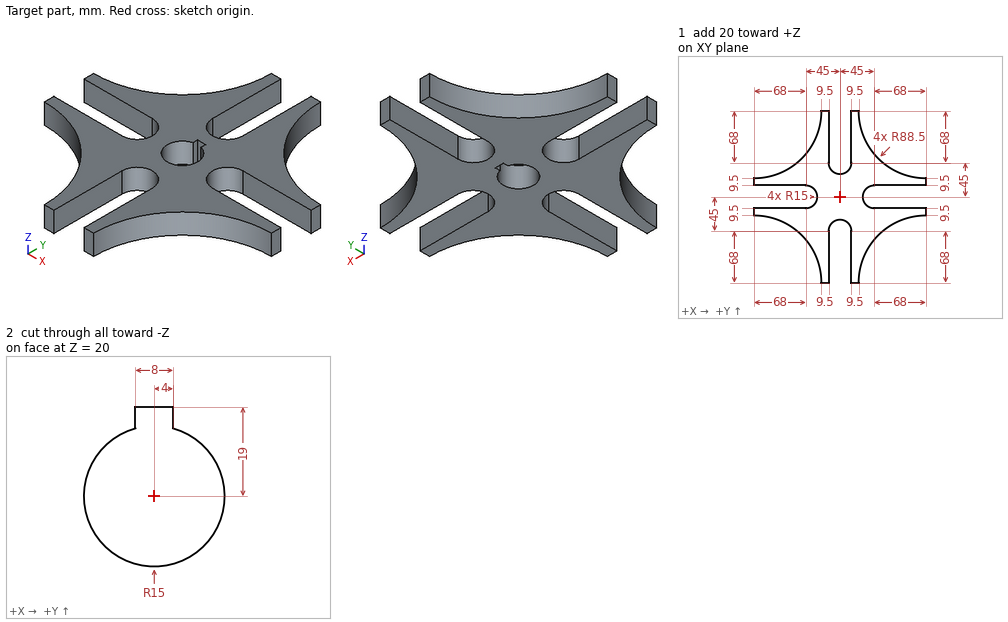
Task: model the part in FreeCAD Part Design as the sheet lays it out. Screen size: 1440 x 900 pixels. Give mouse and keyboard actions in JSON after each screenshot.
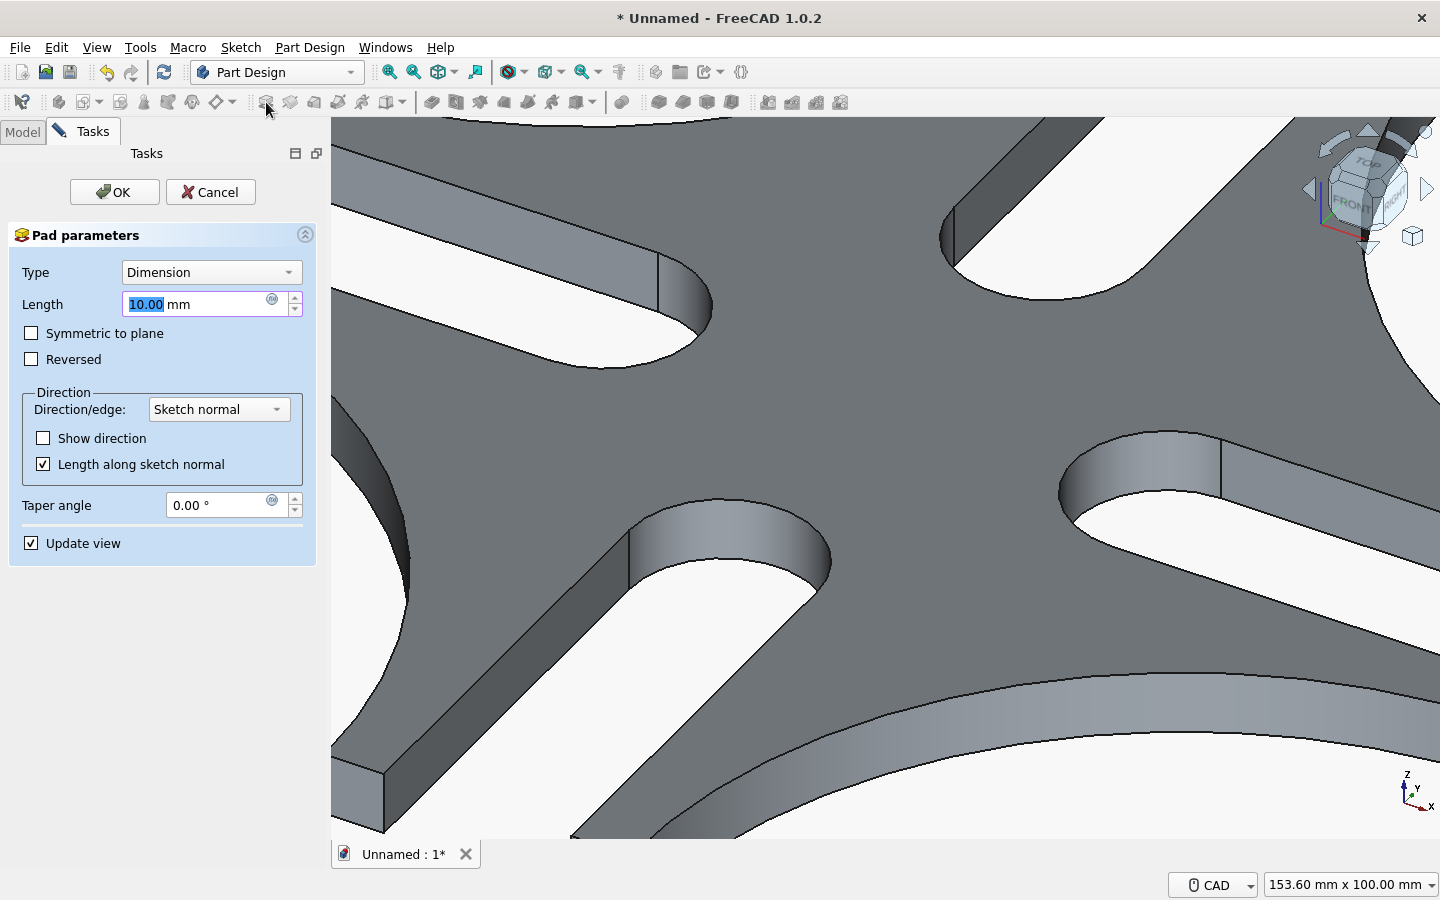
{"action": "type", "text": "20"}
{"action": "key", "text": "Tab"}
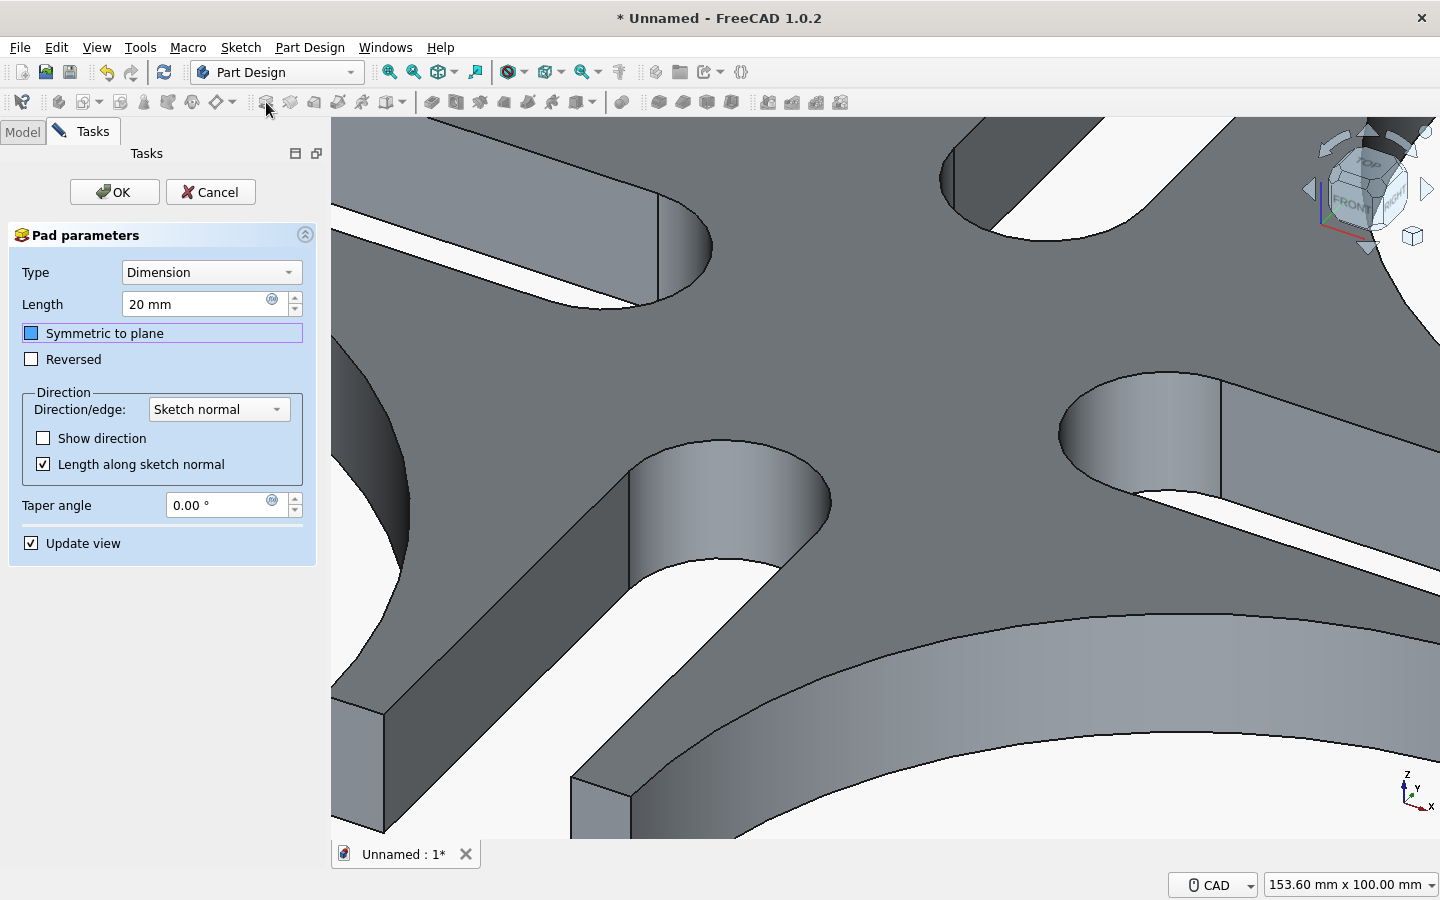
{"action": "left_click", "coordinate": [115, 192]}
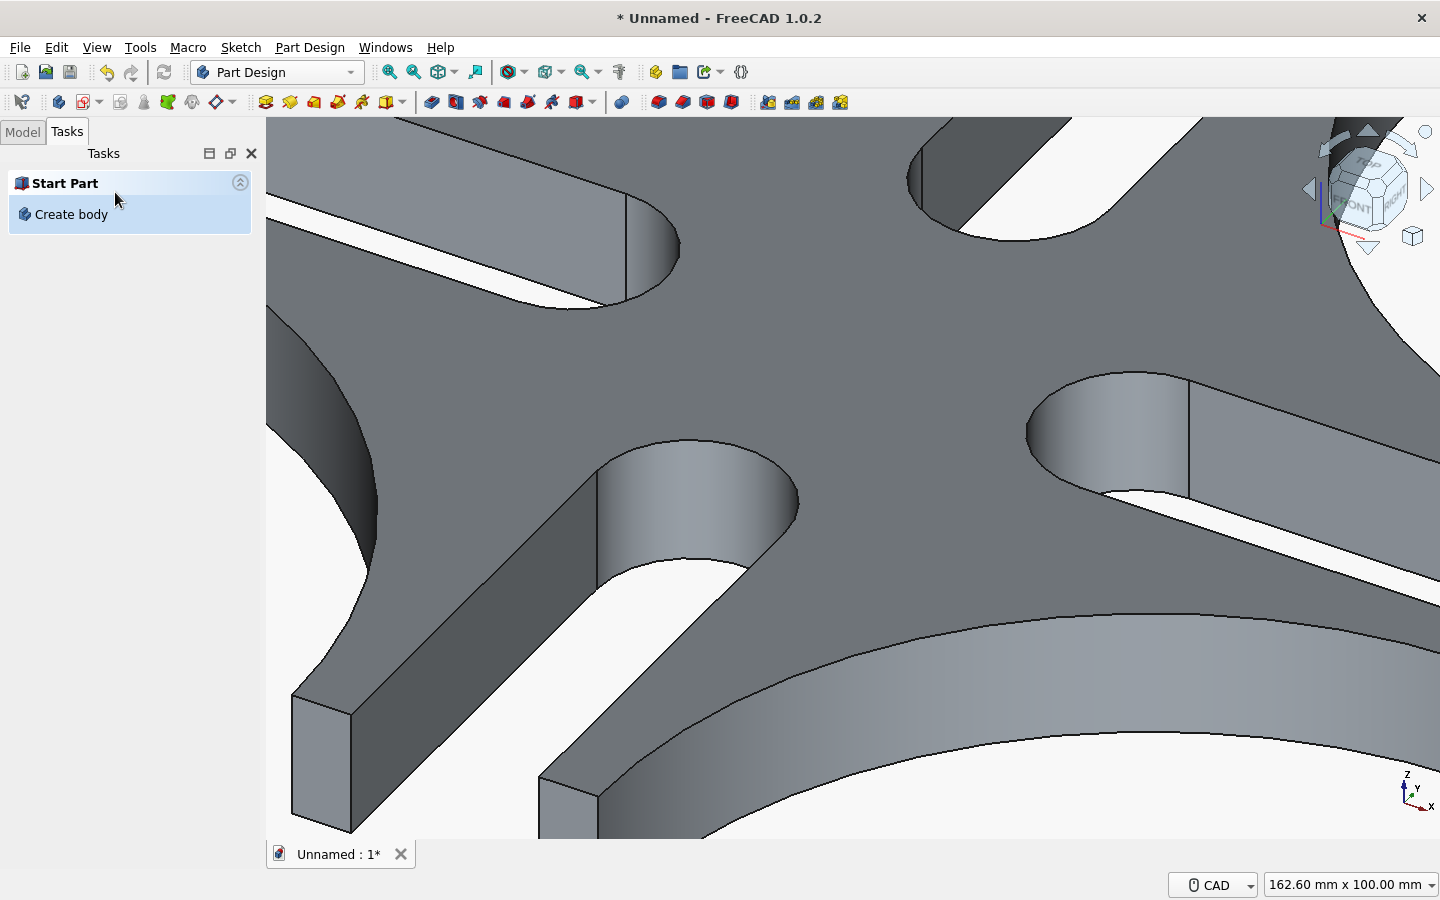
{"action": "left_click", "coordinate": [390, 72]}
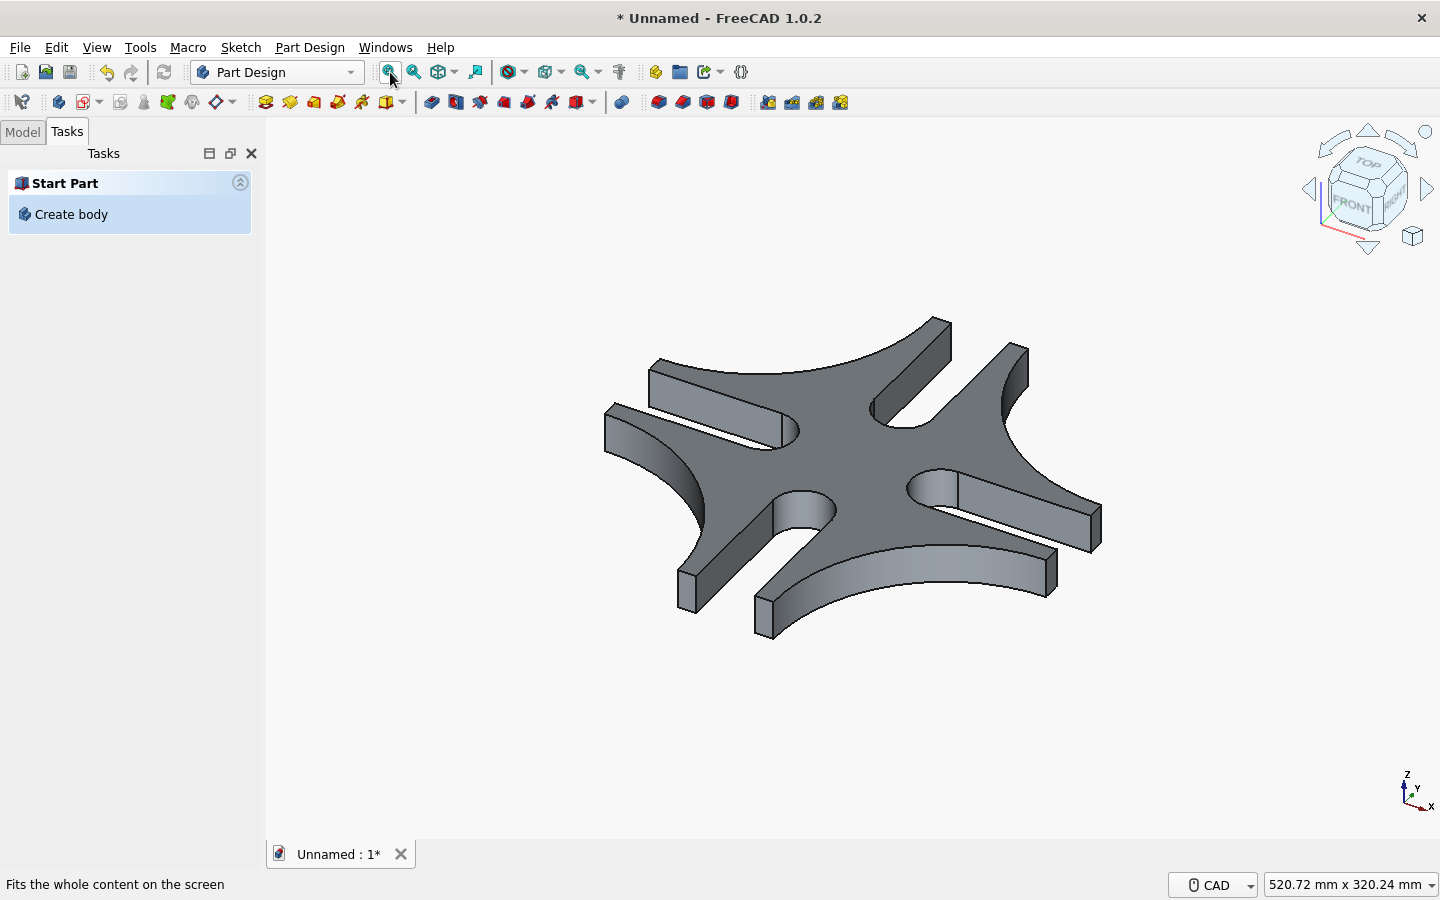
{"action": "left_click", "coordinate": [853, 459]}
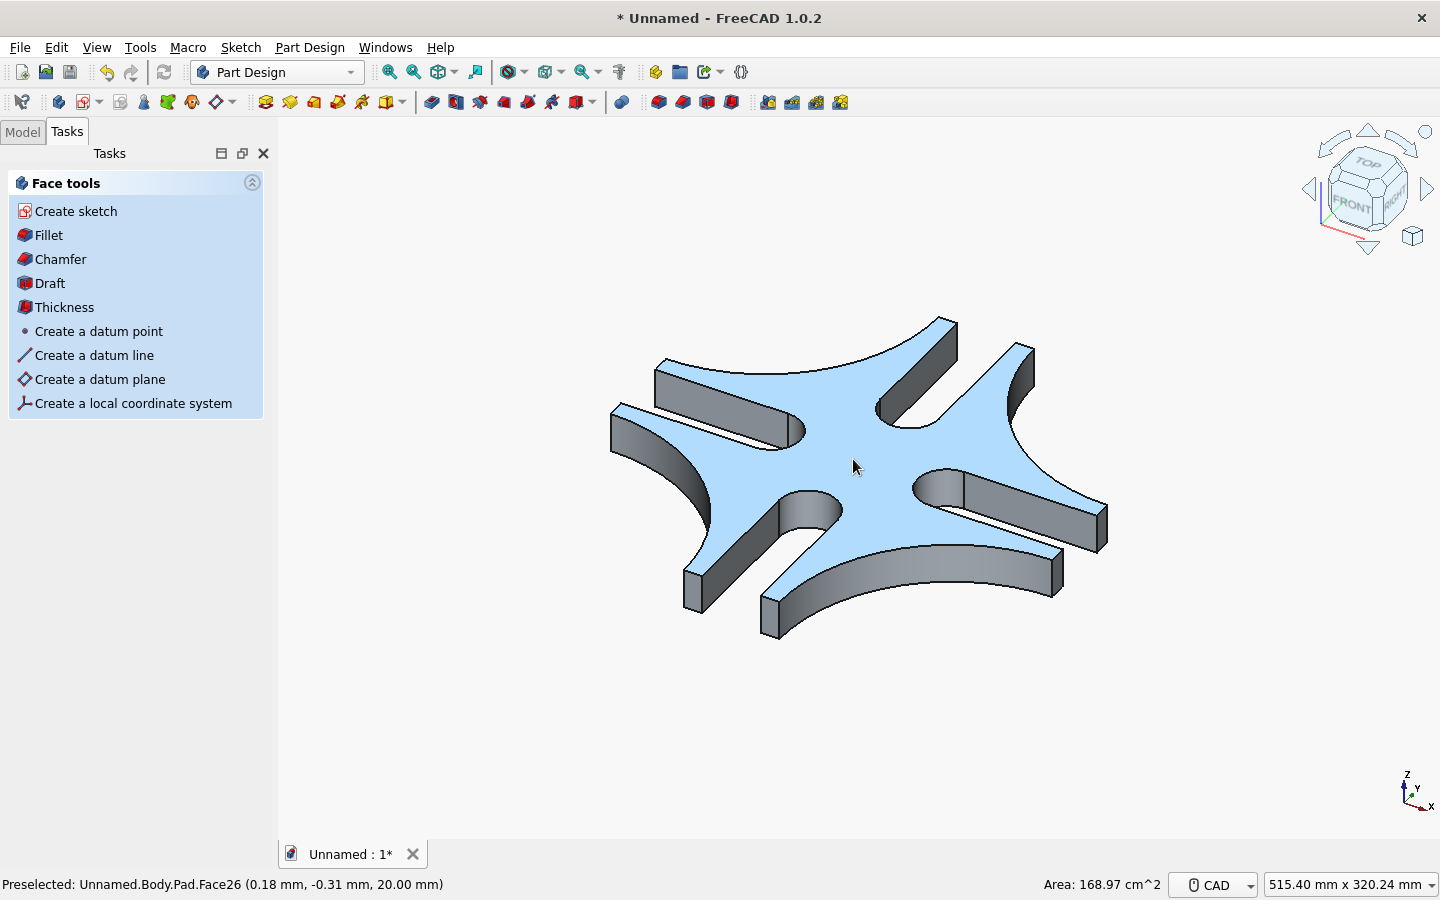
{"action": "left_click", "coordinate": [84, 102]}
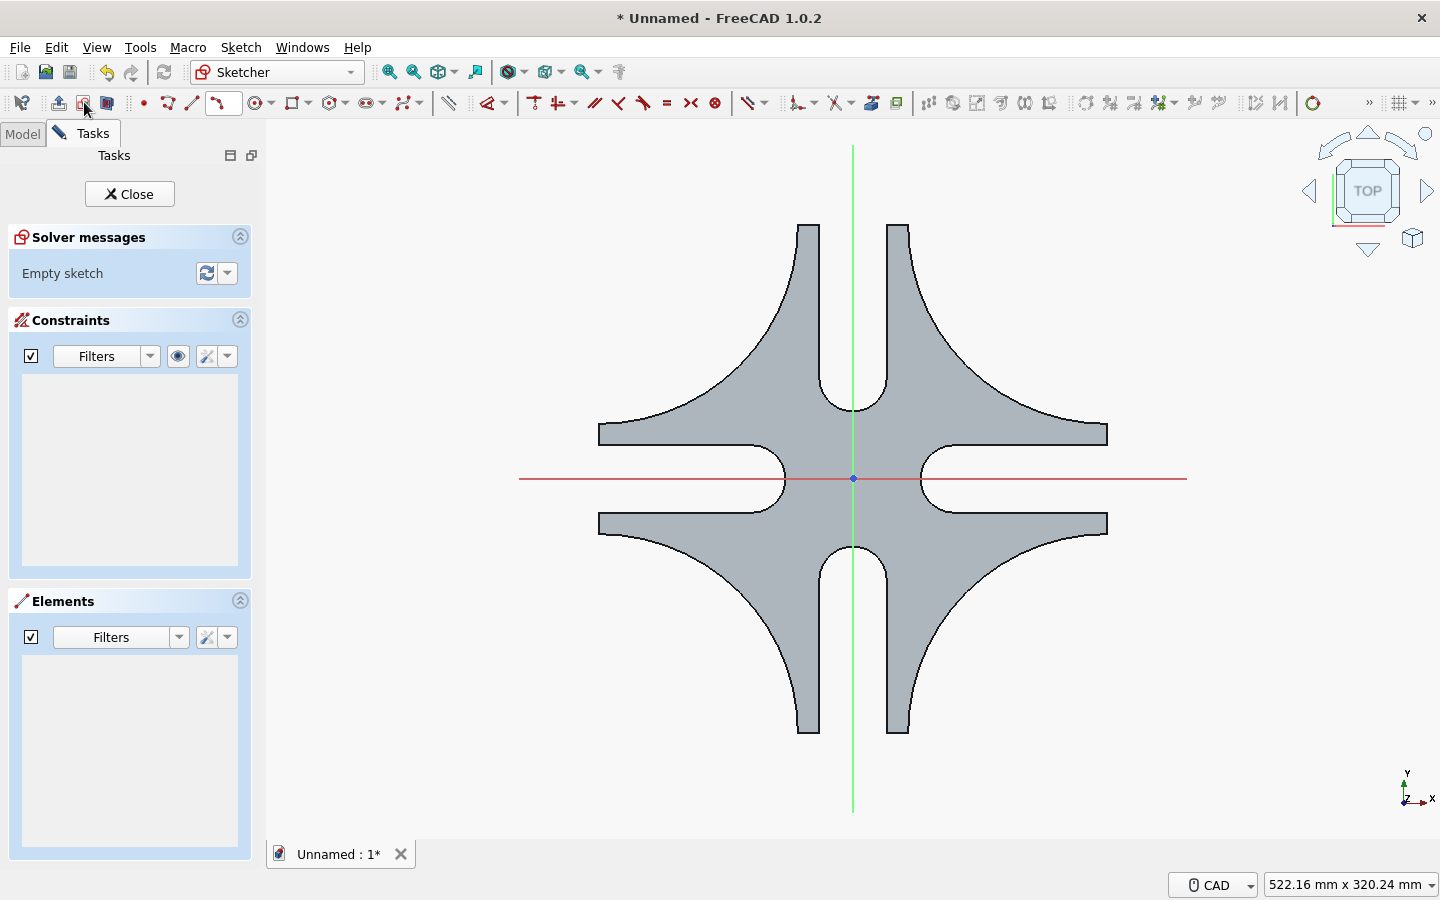
{"action": "scroll", "coordinate": [867, 474], "scroll_direction": "up", "scroll_amount": 9}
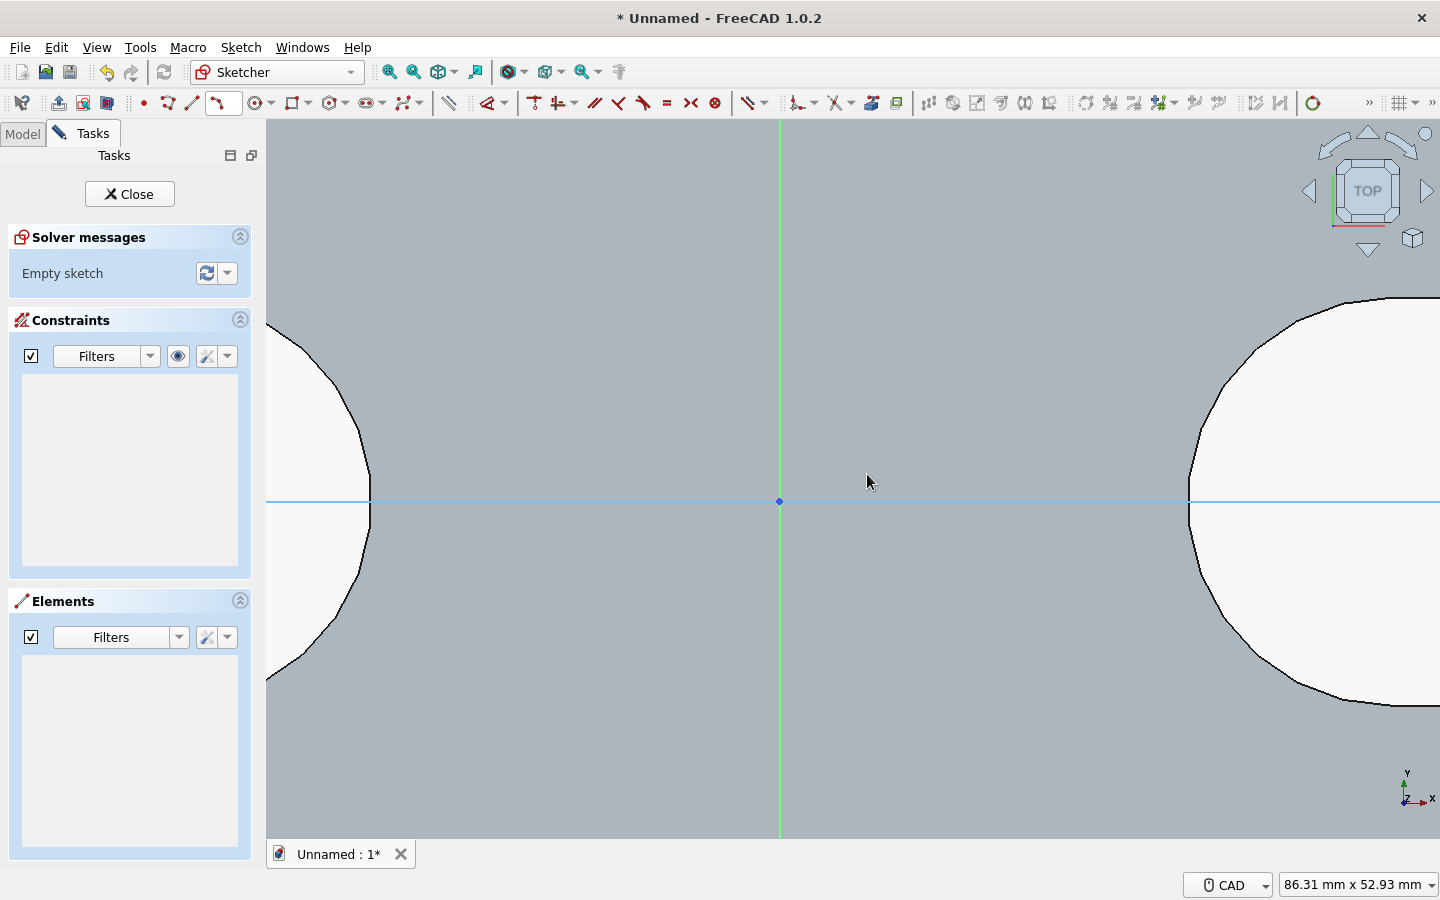
{"action": "left_click", "coordinate": [168, 104]}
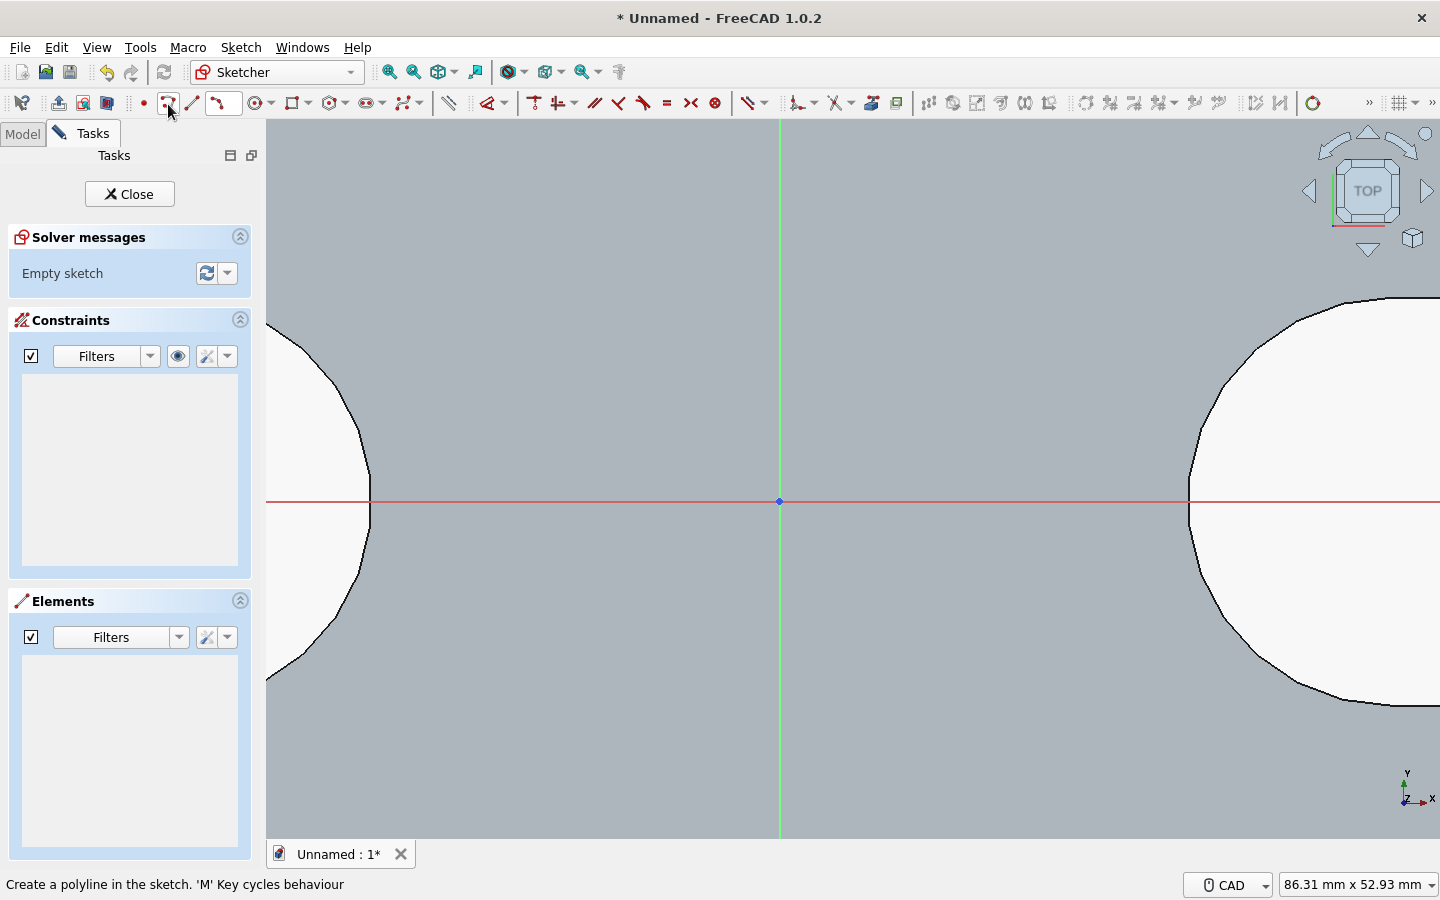
{"action": "left_click", "coordinate": [834, 305]}
{"action": "left_click", "coordinate": [834, 243]}
{"action": "left_click", "coordinate": [725, 243]}
{"action": "left_click", "coordinate": [725, 305]}
{"action": "right_click", "coordinate": [725, 305]}